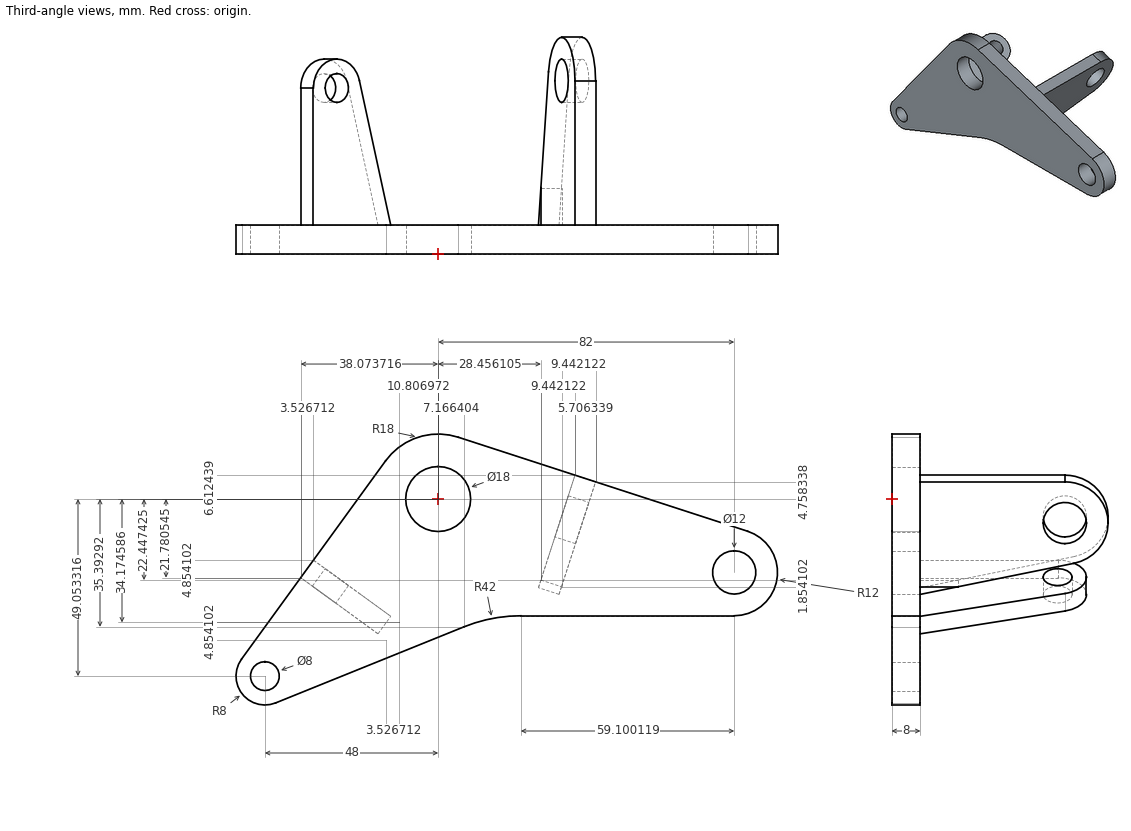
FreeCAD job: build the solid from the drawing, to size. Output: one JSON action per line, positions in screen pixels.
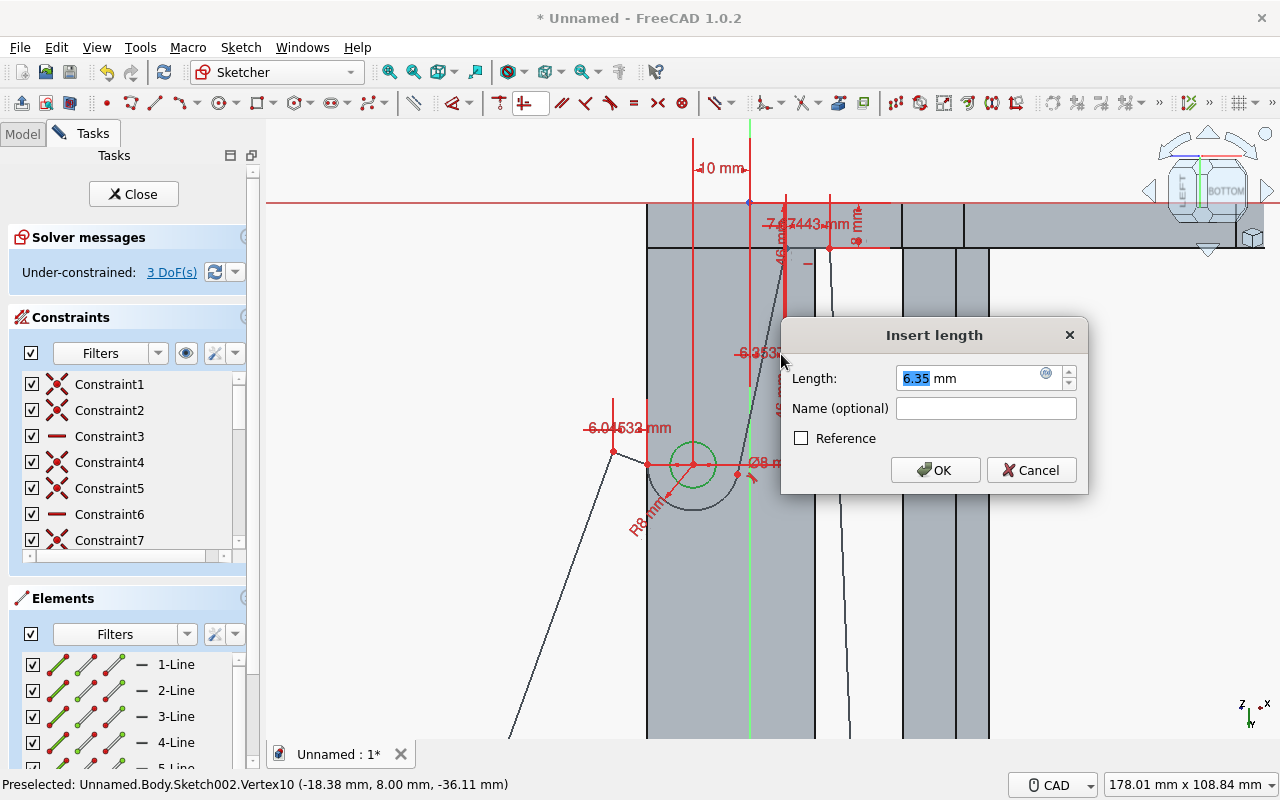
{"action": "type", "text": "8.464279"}
{"action": "key", "text": "Return"}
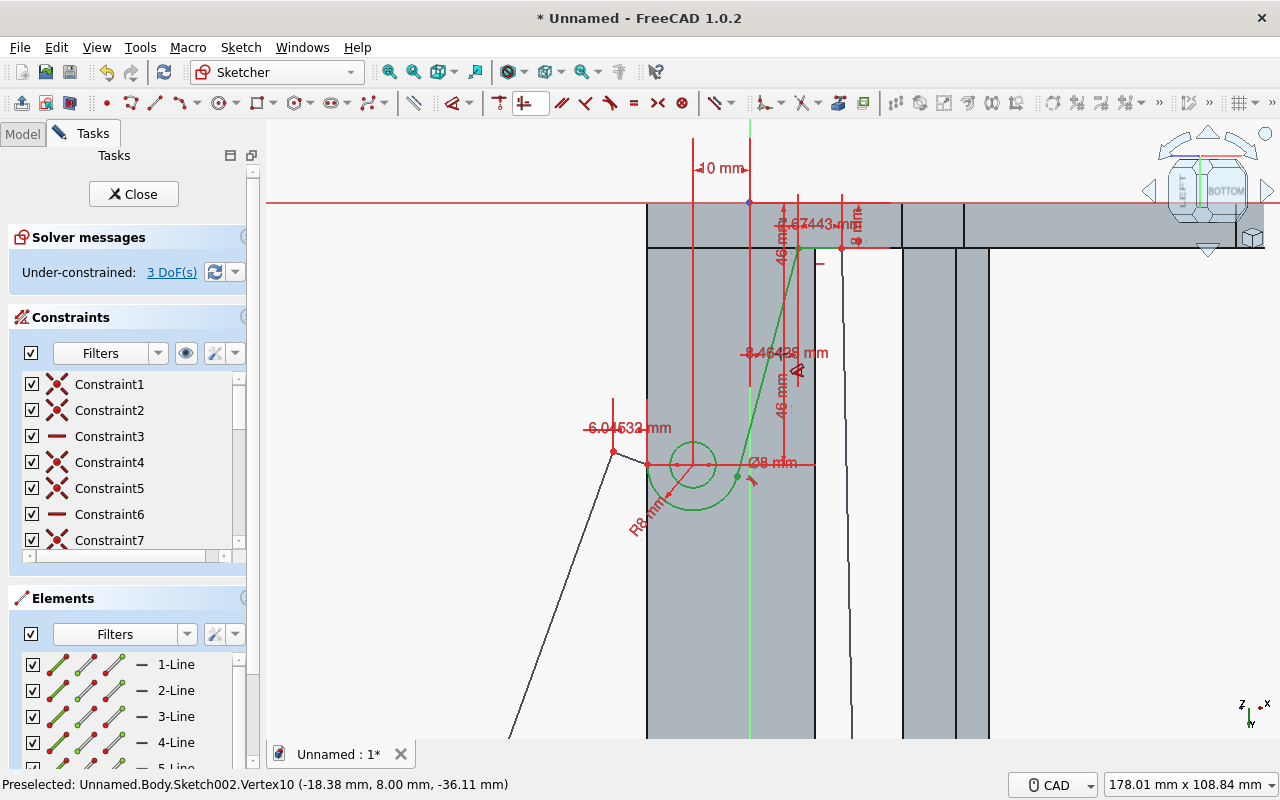
{"action": "scroll", "coordinate": [637, 461], "scroll_direction": "up", "scroll_amount": 5}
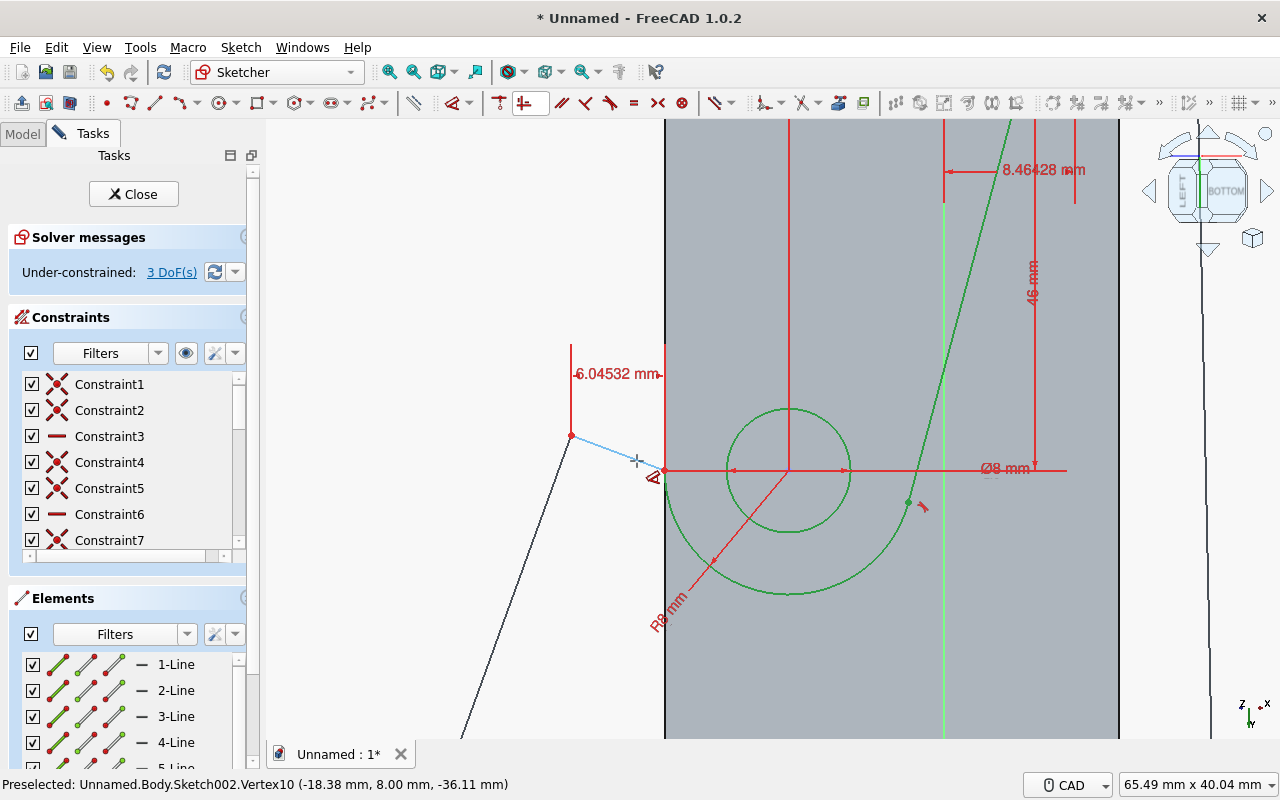
{"action": "left_click", "coordinate": [637, 460]}
{"action": "left_click", "coordinate": [537, 453]}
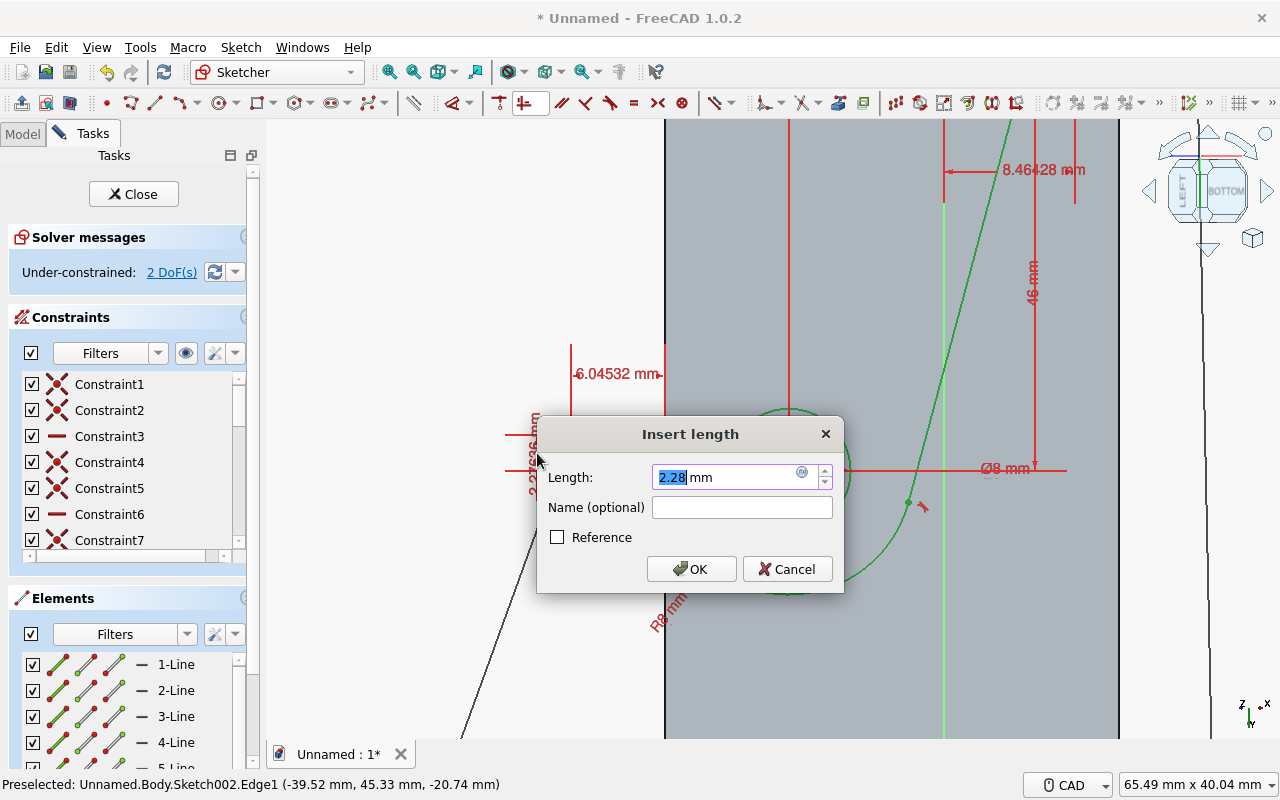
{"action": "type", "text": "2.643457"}
{"action": "key", "text": "Return"}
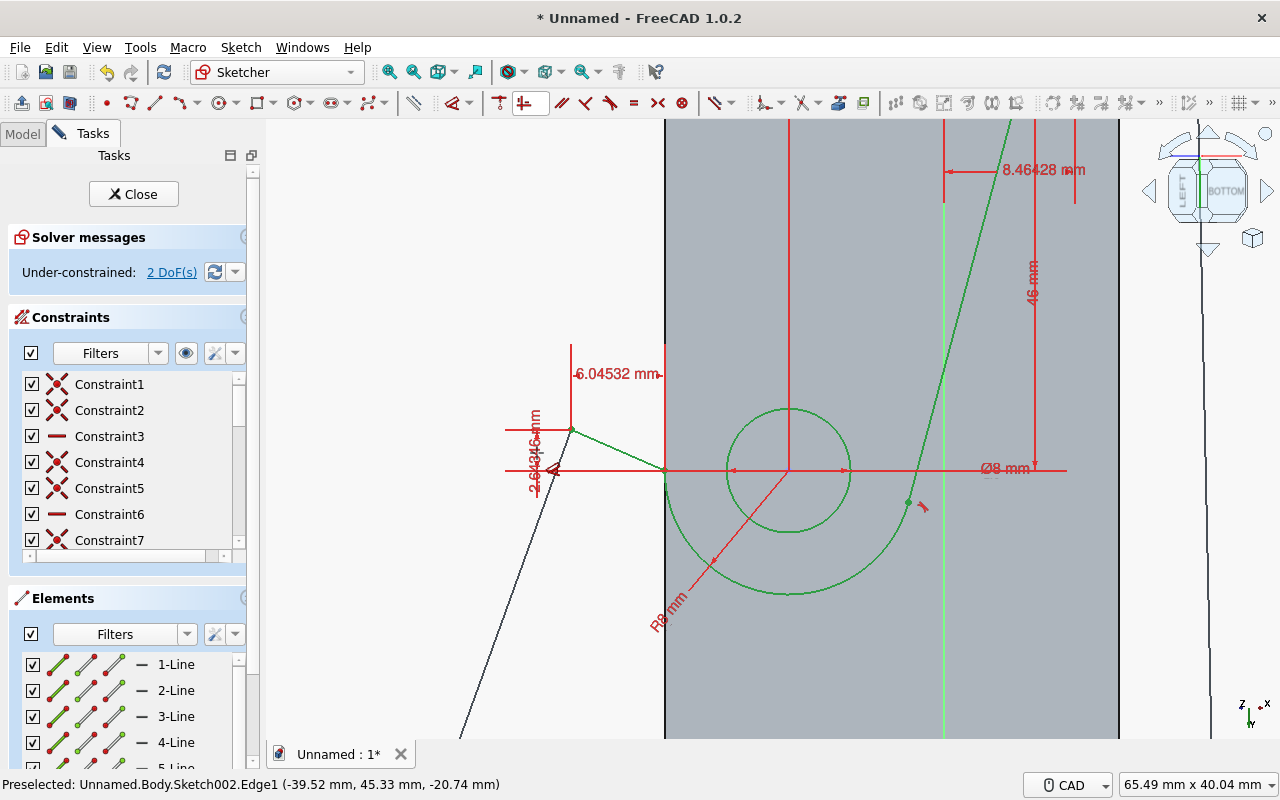
{"action": "scroll", "coordinate": [703, 368], "scroll_direction": "down", "scroll_amount": 7}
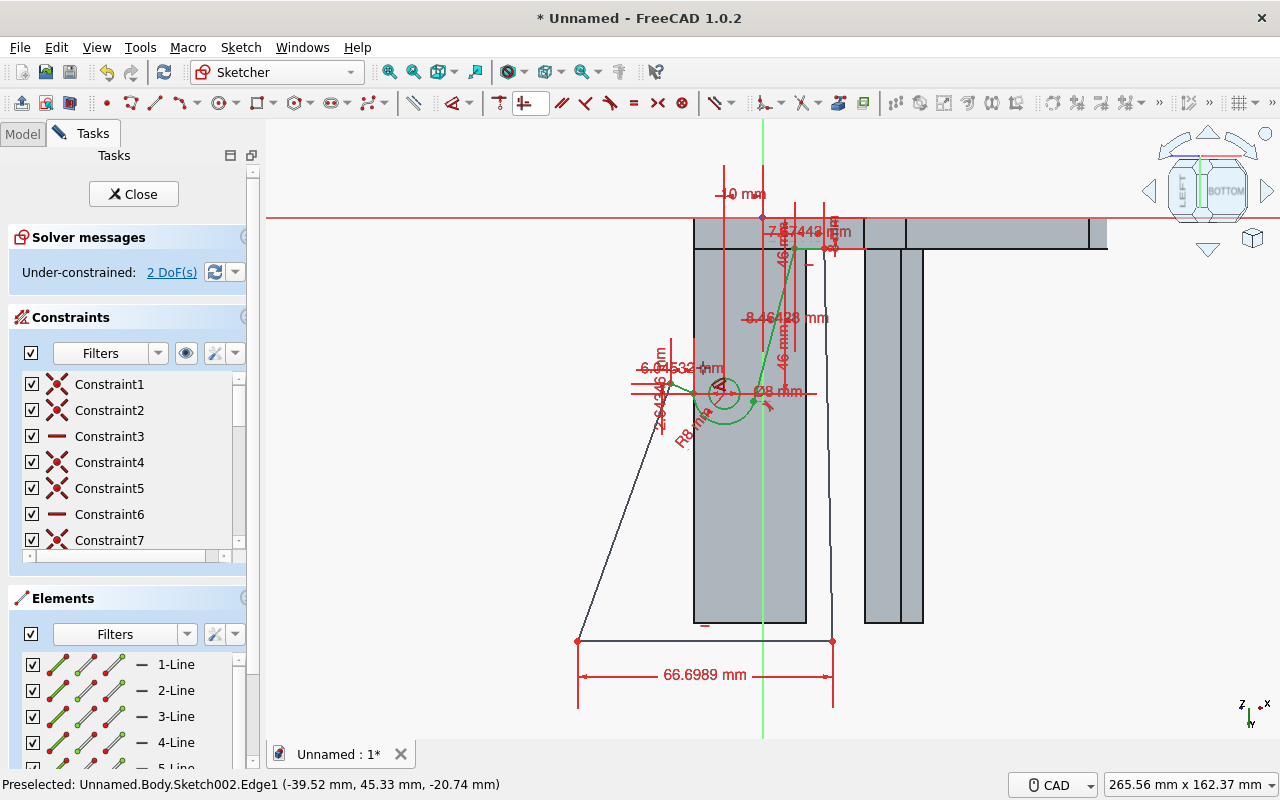
{"action": "scroll", "coordinate": [830, 524], "scroll_direction": "up", "scroll_amount": 8}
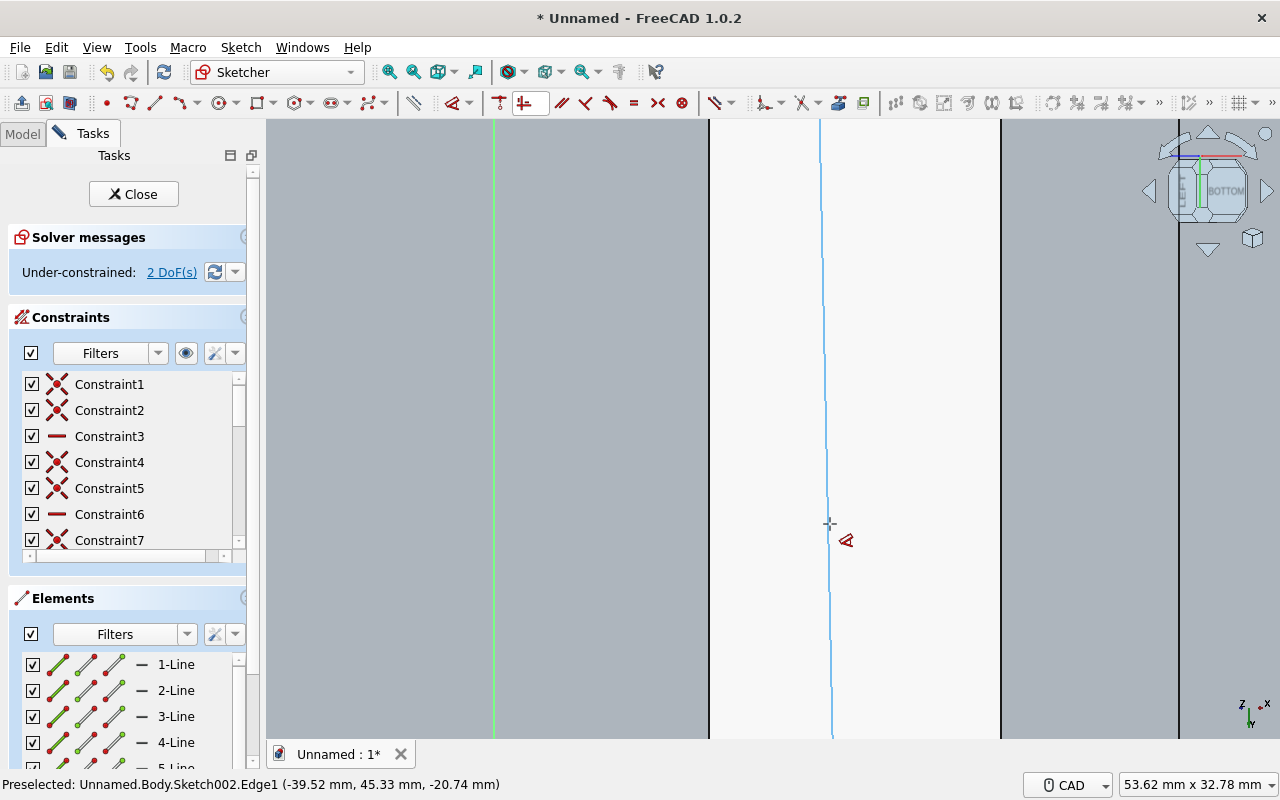
{"action": "left_click", "coordinate": [828, 519]}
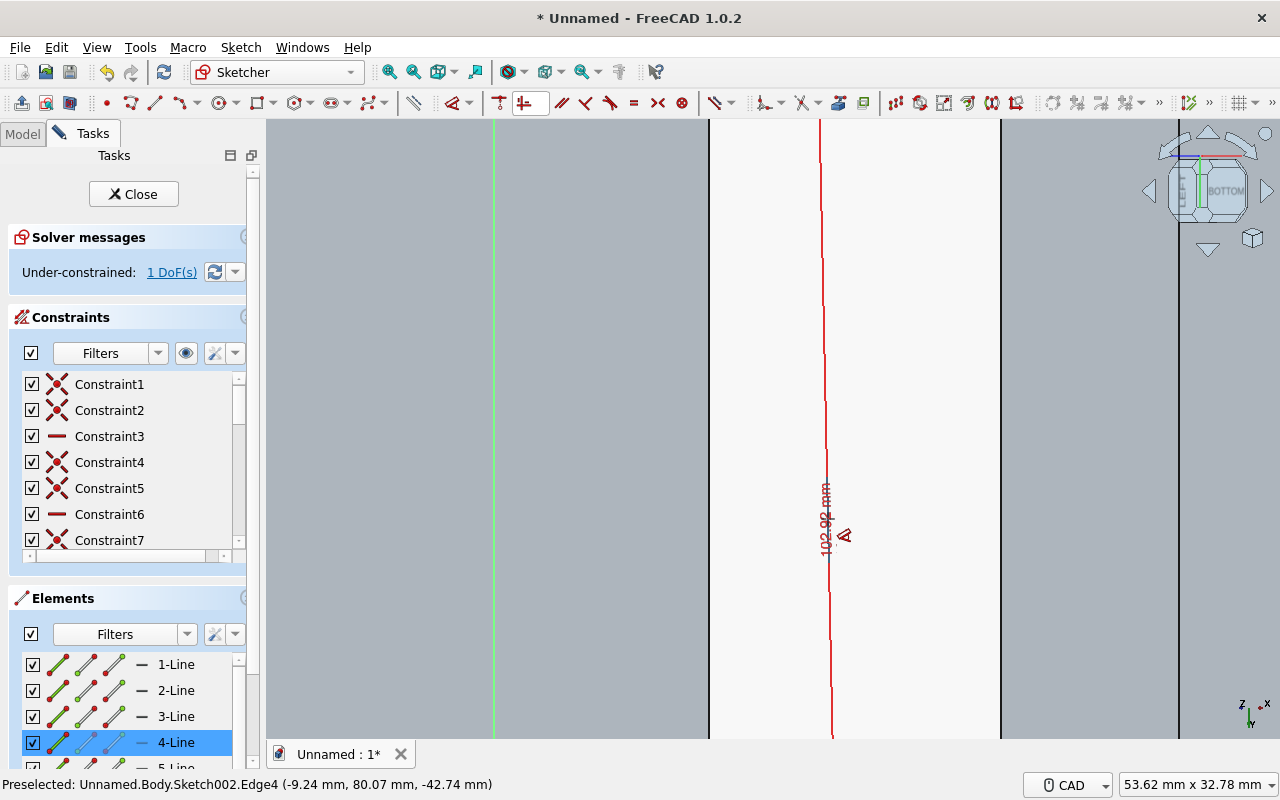
{"action": "key", "text": "Escape"}
{"action": "key", "text": "Escape"}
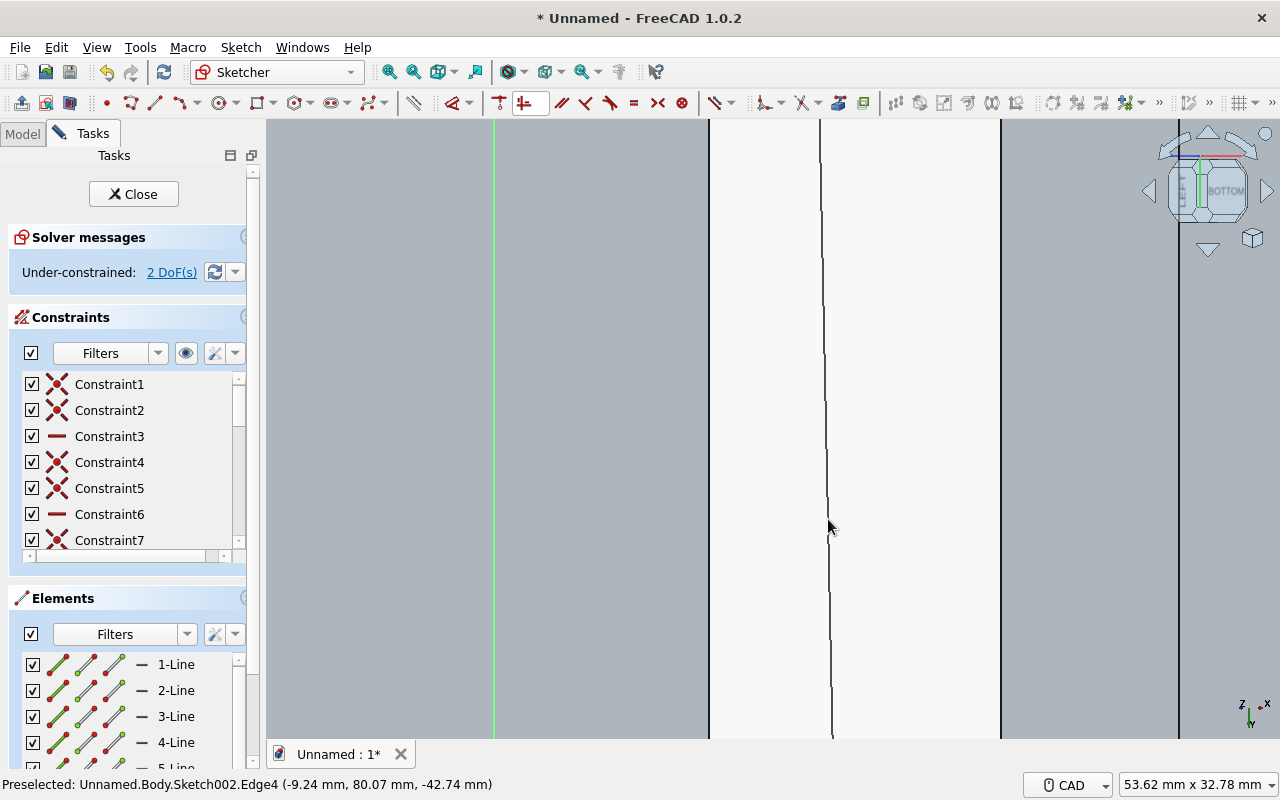
{"action": "left_click", "coordinate": [828, 519]}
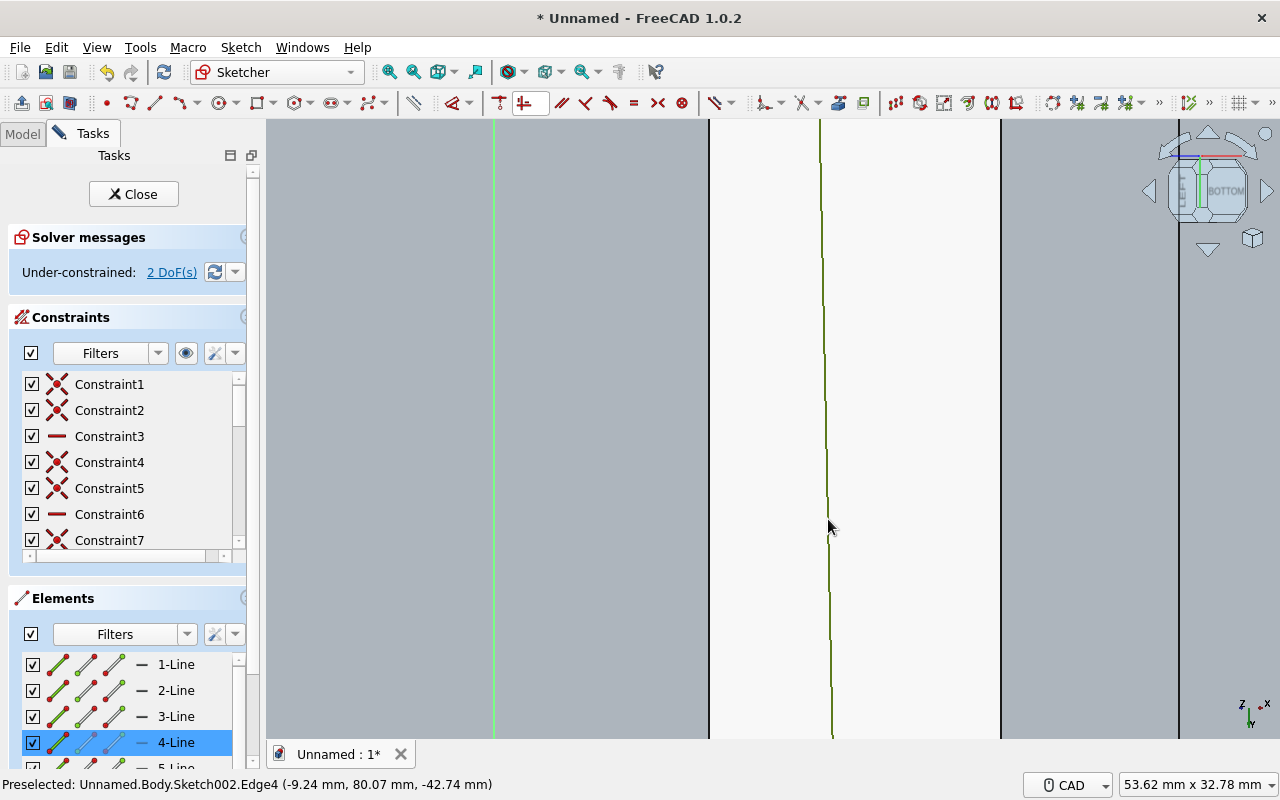
{"action": "left_click", "coordinate": [472, 104]}